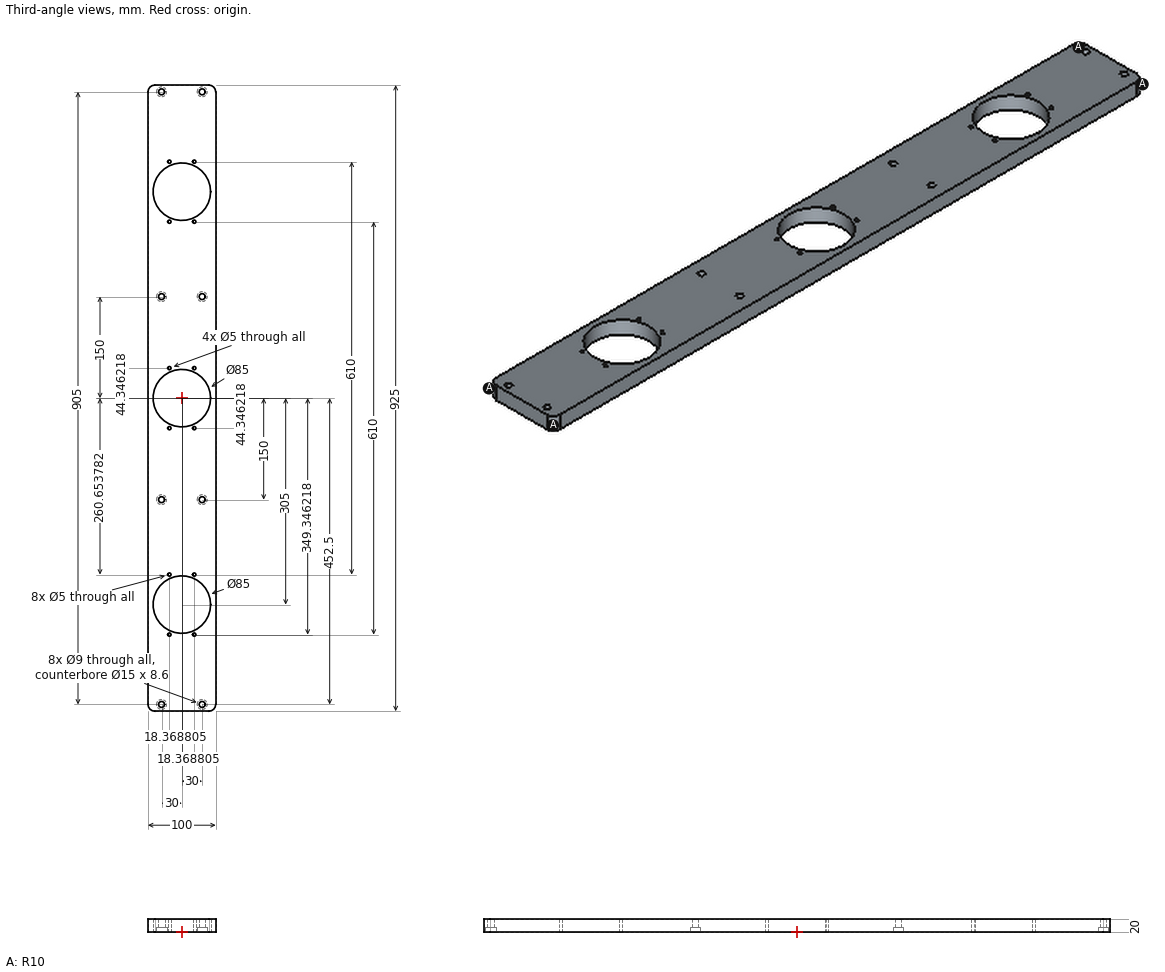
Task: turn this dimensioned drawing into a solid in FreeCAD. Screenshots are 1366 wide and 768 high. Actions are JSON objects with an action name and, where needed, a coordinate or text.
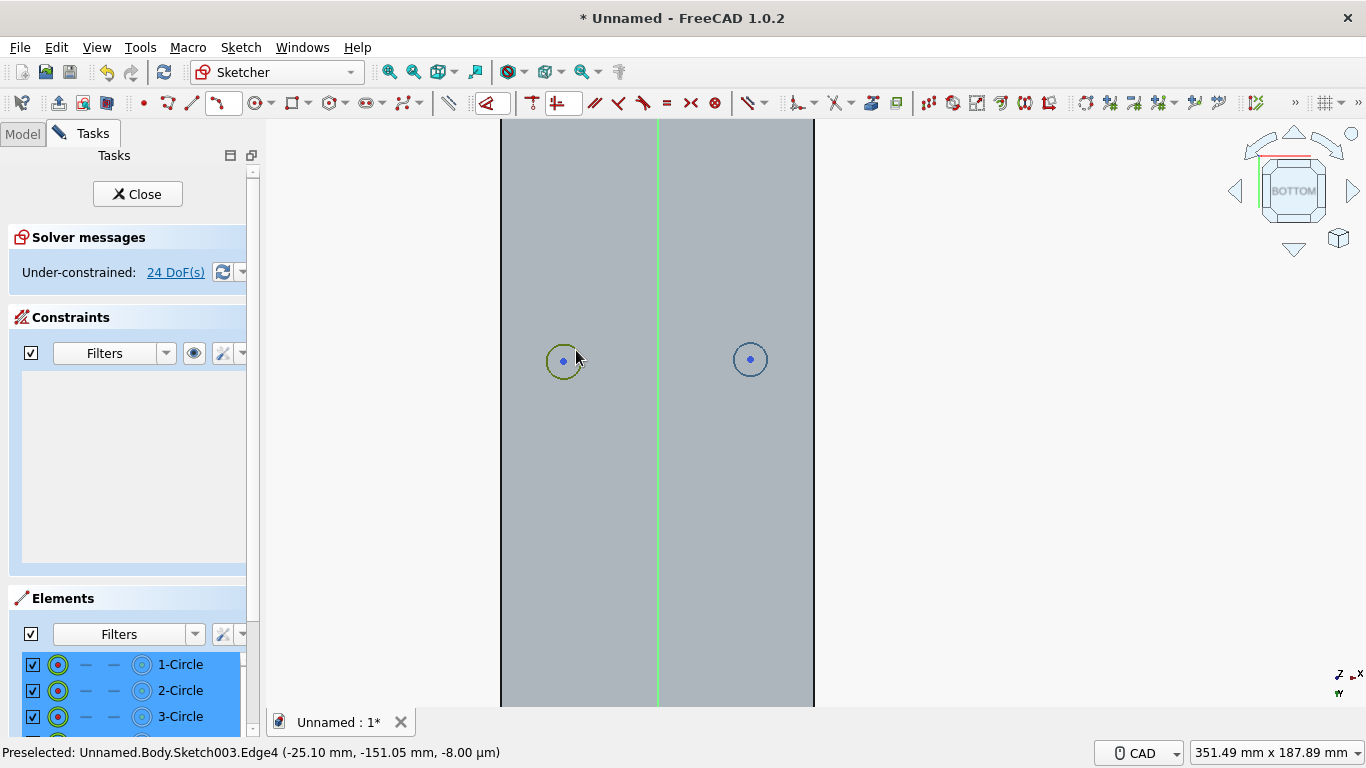
{"action": "scroll", "coordinate": [762, 348], "scroll_direction": "down", "scroll_amount": 10}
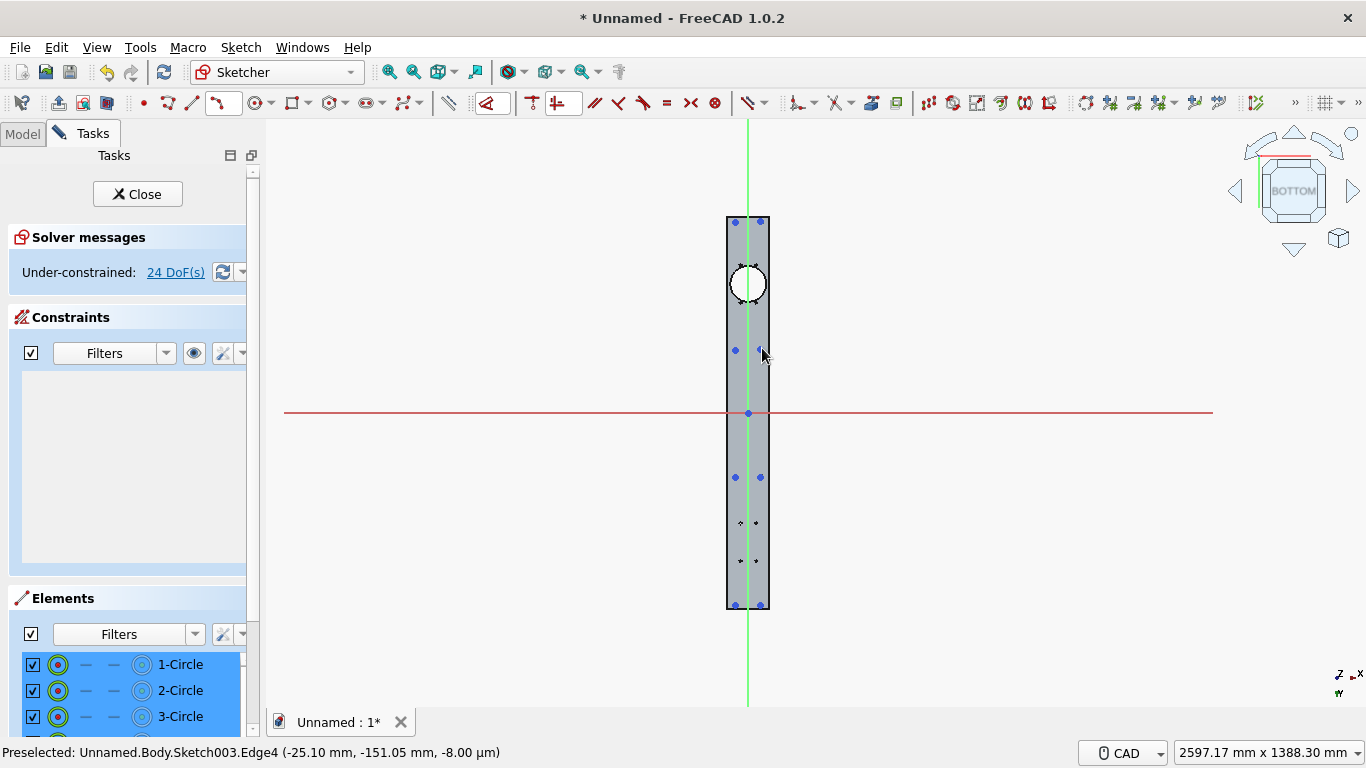
{"action": "scroll", "coordinate": [737, 476], "scroll_direction": "up", "scroll_amount": 10}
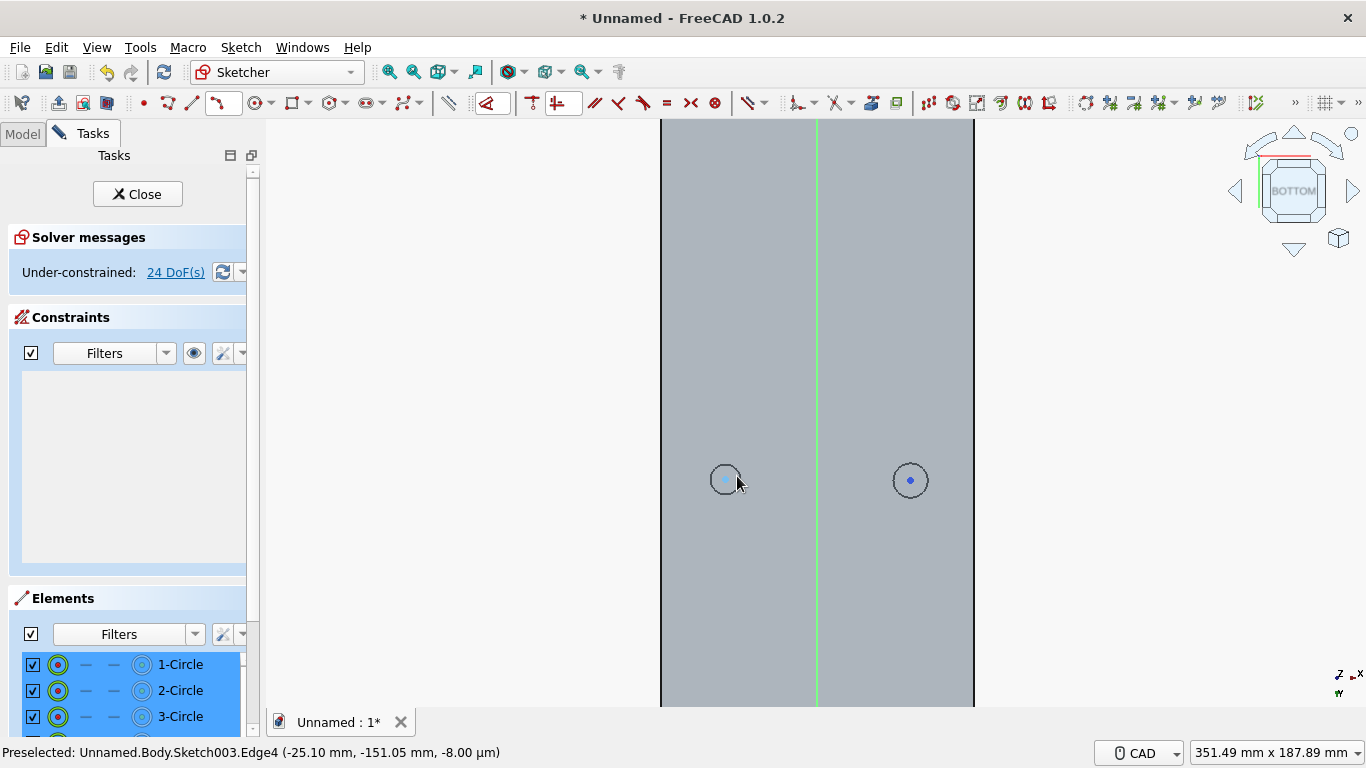
{"action": "left_click", "coordinate": [736, 469]}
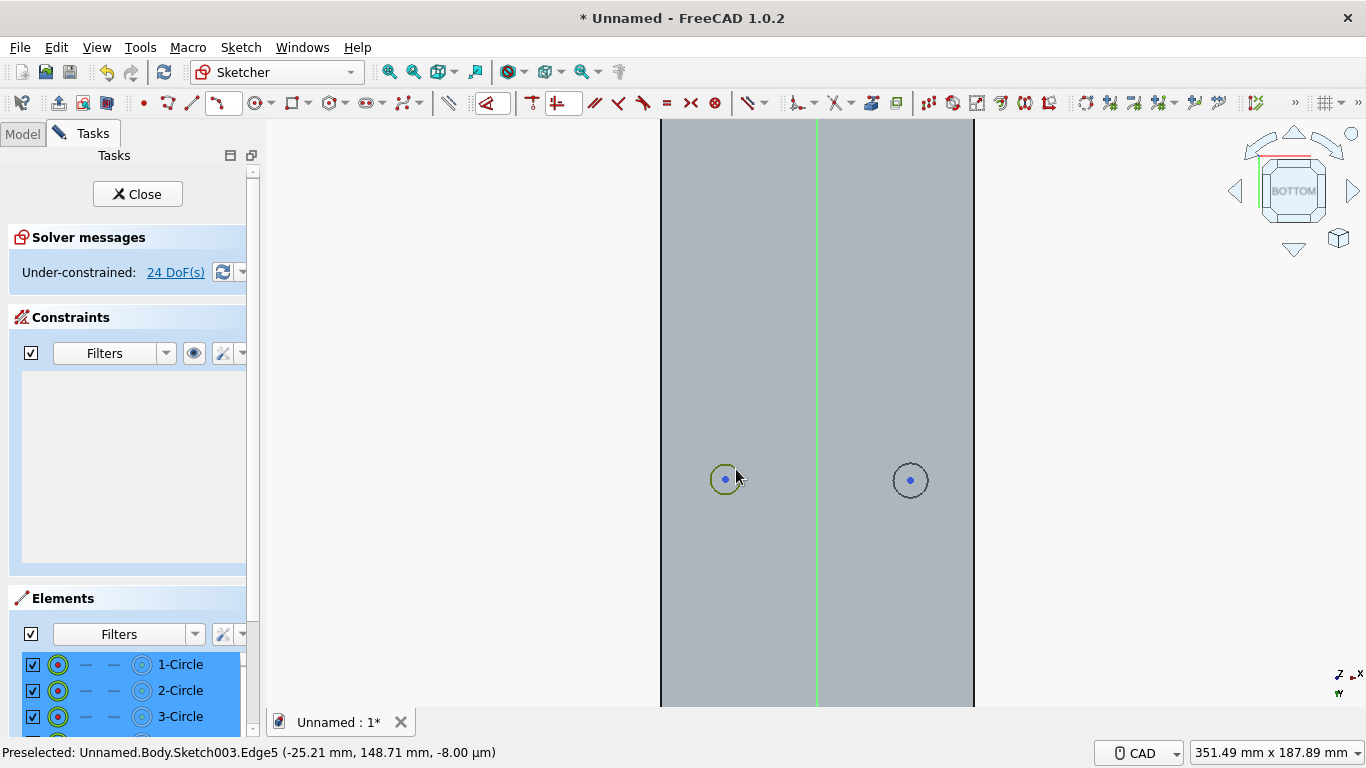
{"action": "left_click", "coordinate": [923, 468]}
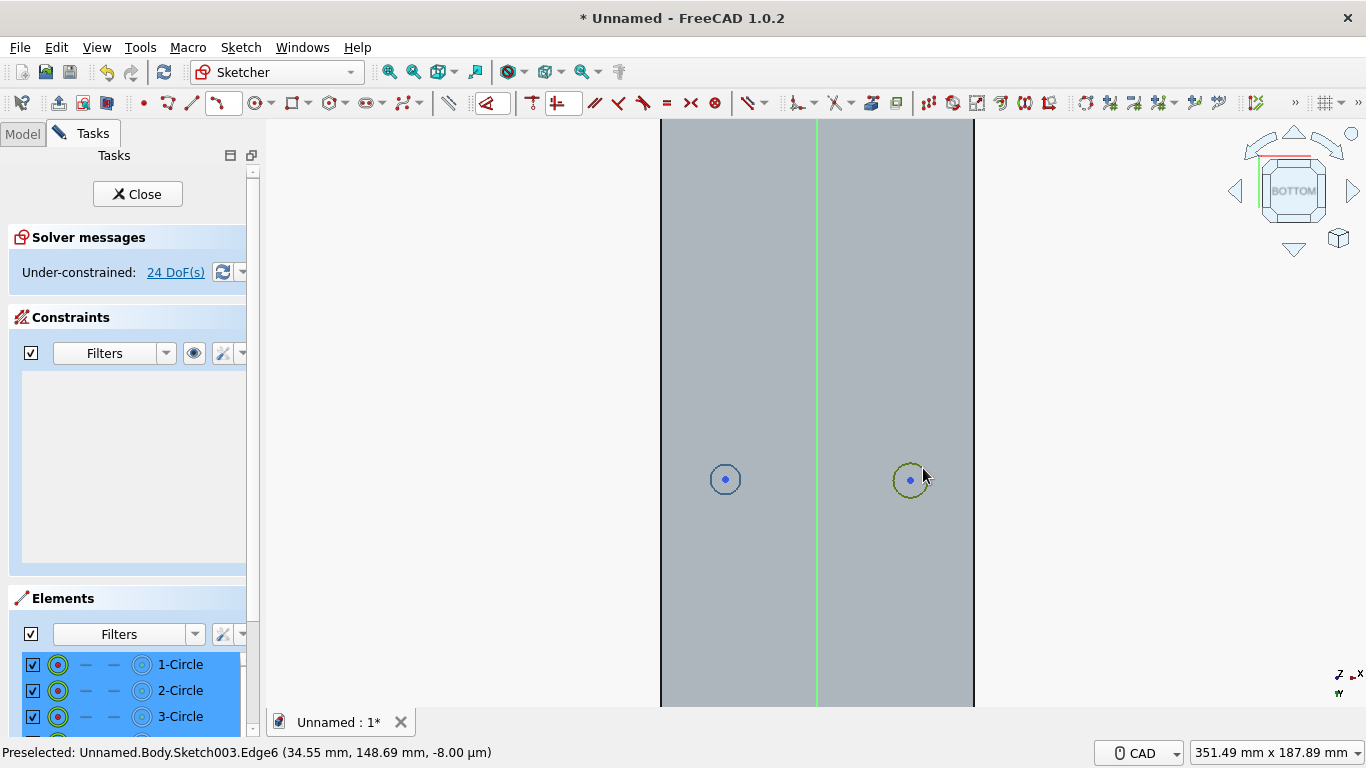
{"action": "scroll", "coordinate": [737, 477], "scroll_direction": "down", "scroll_amount": 10}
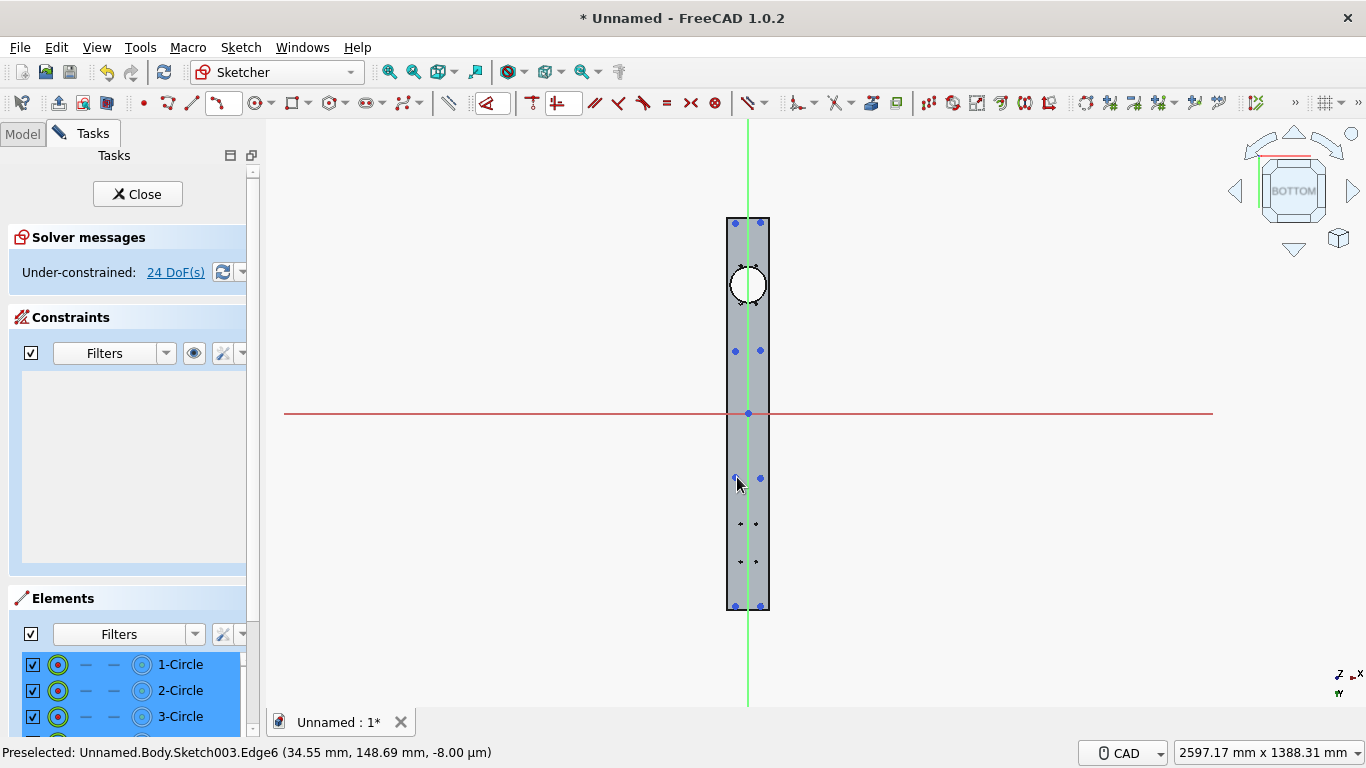
{"action": "scroll", "coordinate": [737, 605], "scroll_direction": "up", "scroll_amount": 10}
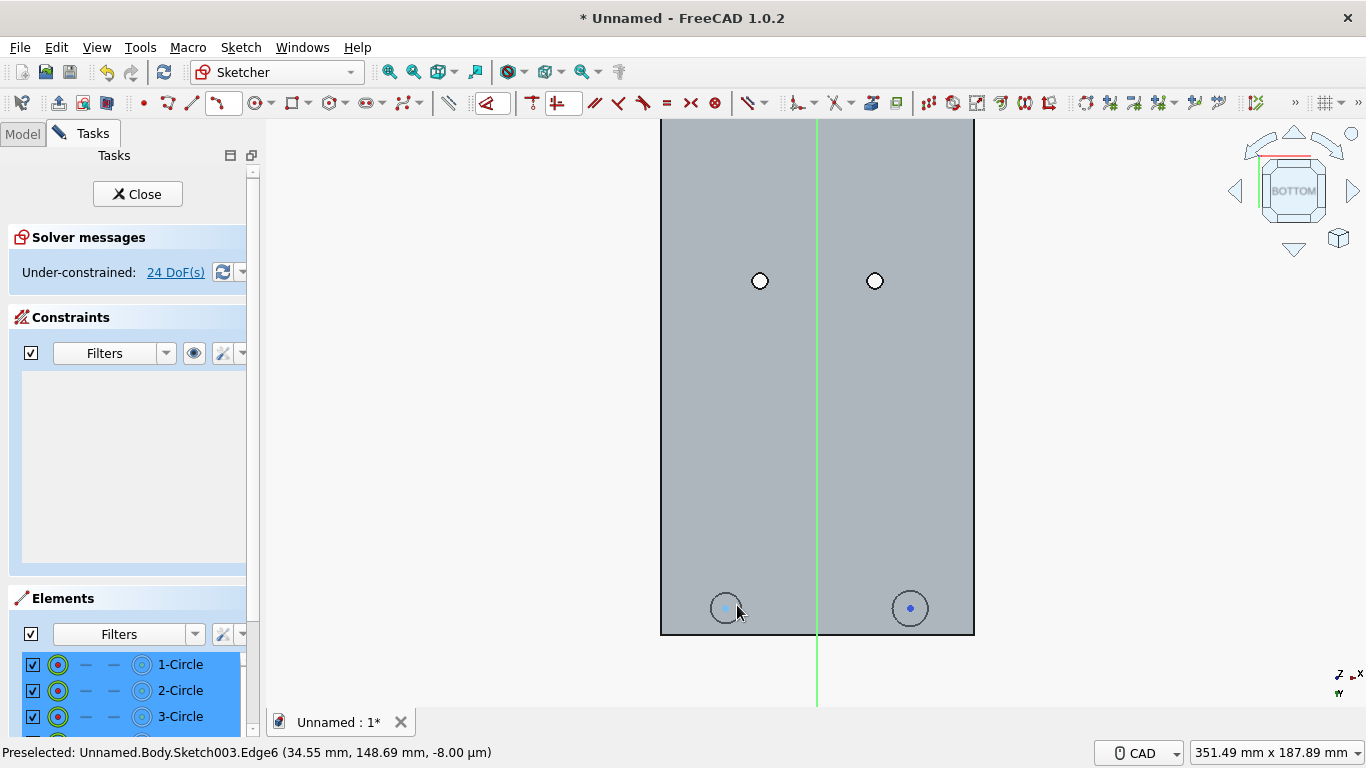
{"action": "left_click", "coordinate": [737, 597]}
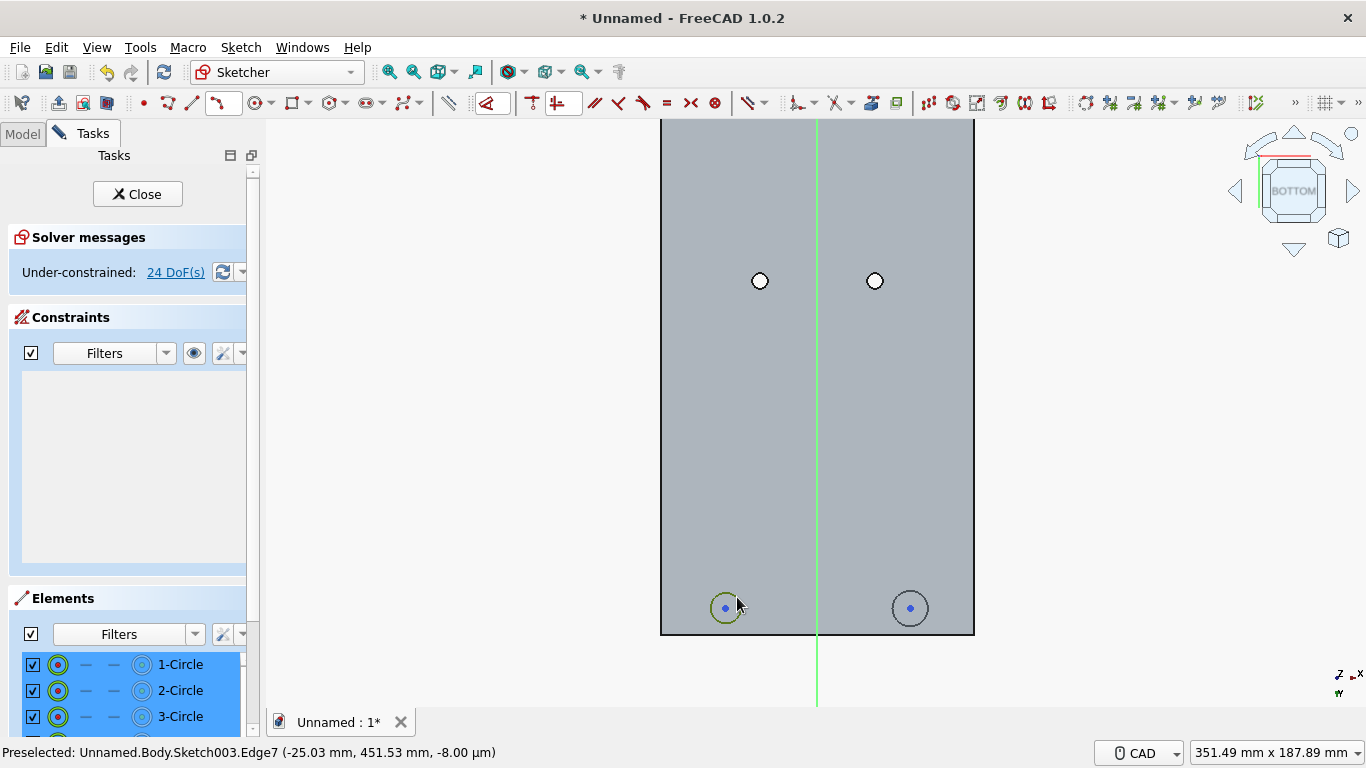
{"action": "left_click", "coordinate": [923, 596]}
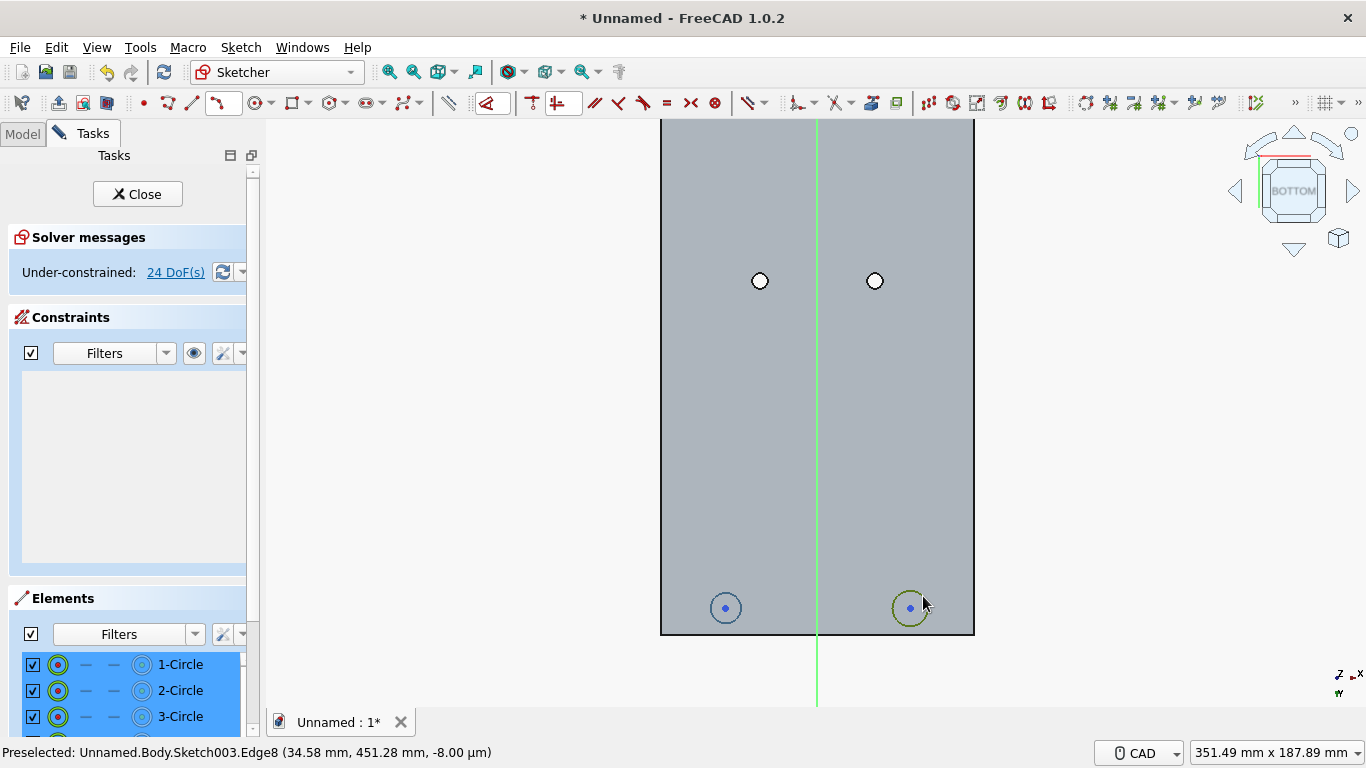
{"action": "key", "text": "e"}